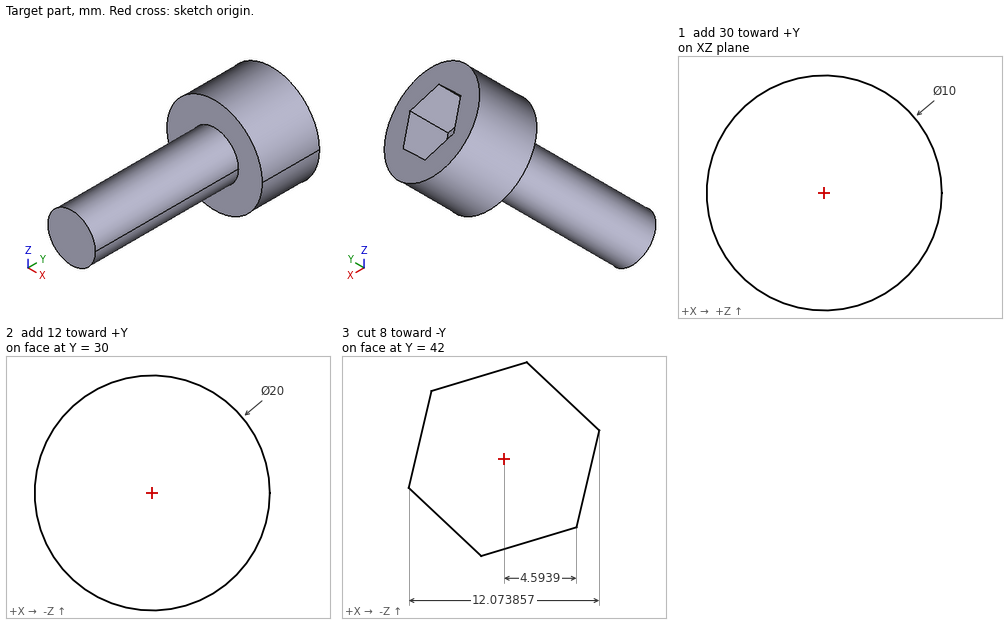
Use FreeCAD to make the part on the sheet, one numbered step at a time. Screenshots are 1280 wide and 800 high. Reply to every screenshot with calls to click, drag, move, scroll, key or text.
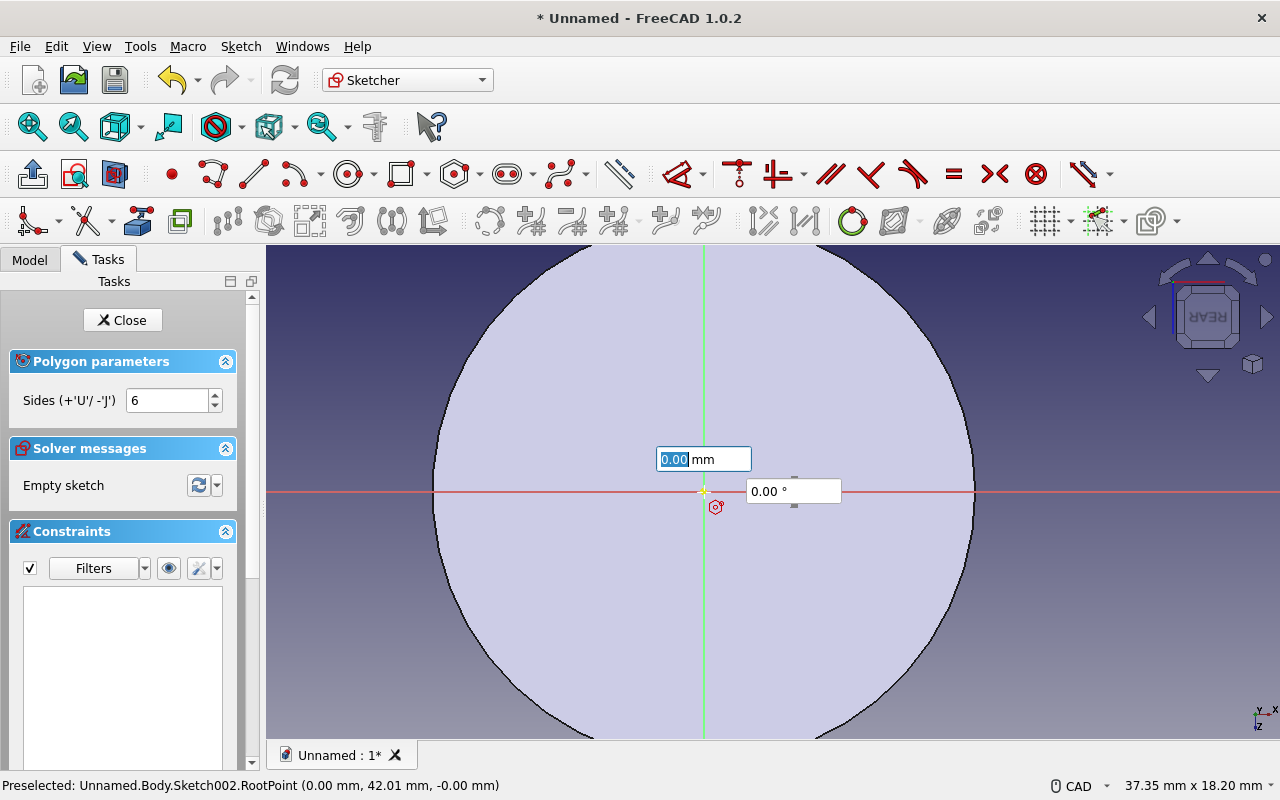
click(829, 609)
right_click(829, 609)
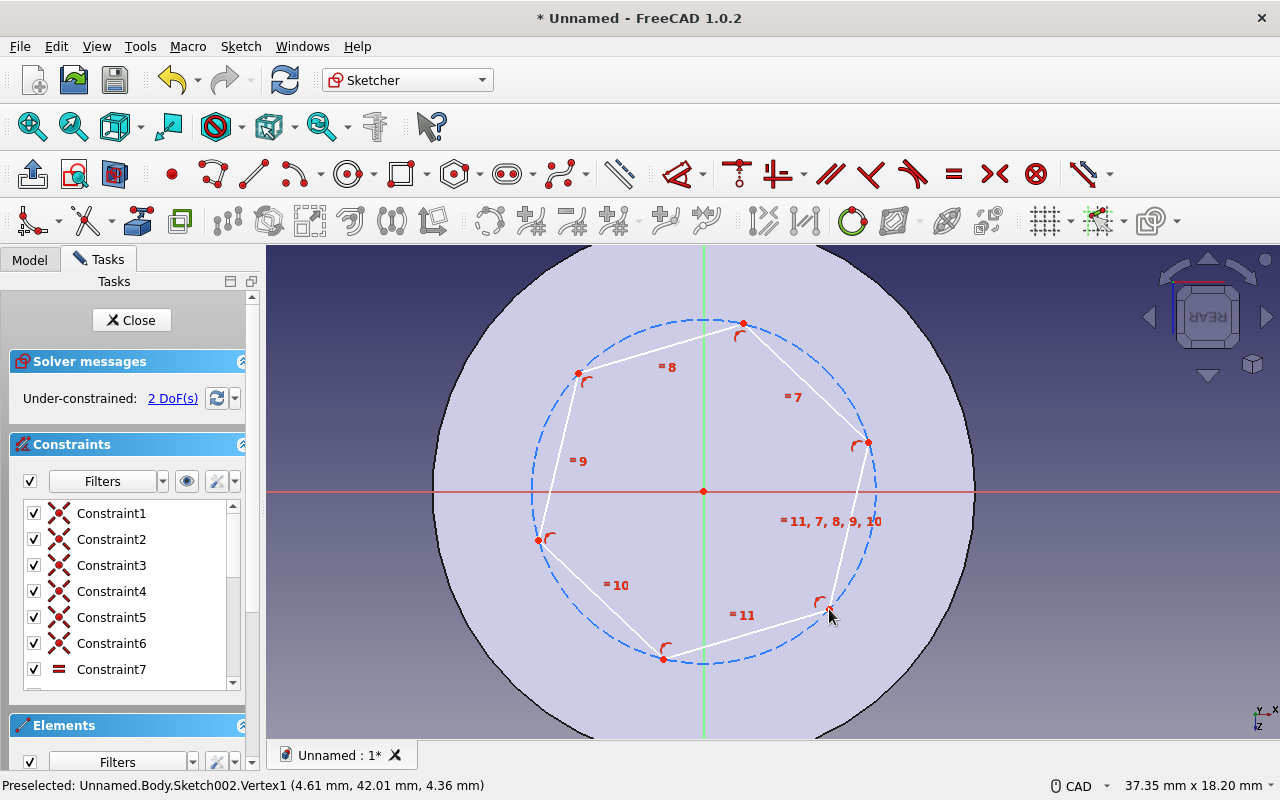
key(d)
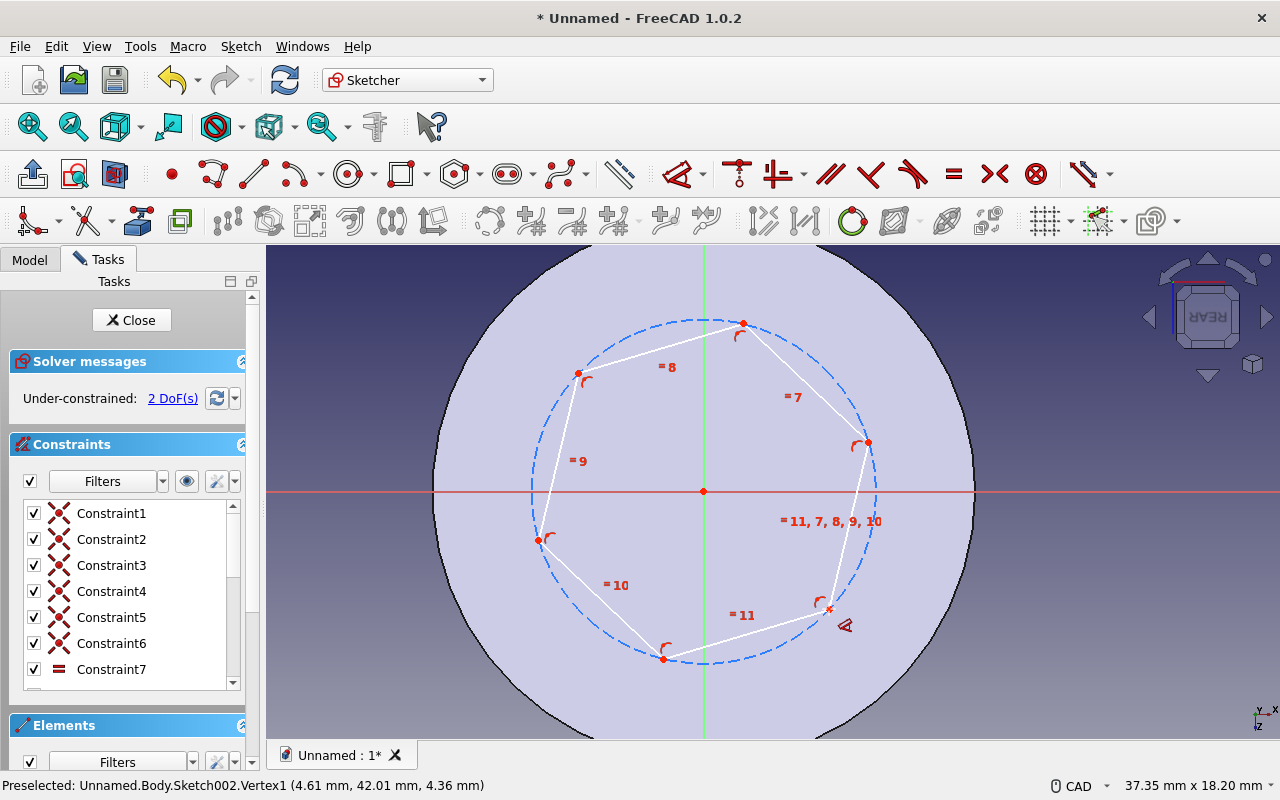
click(829, 610)
click(810, 644)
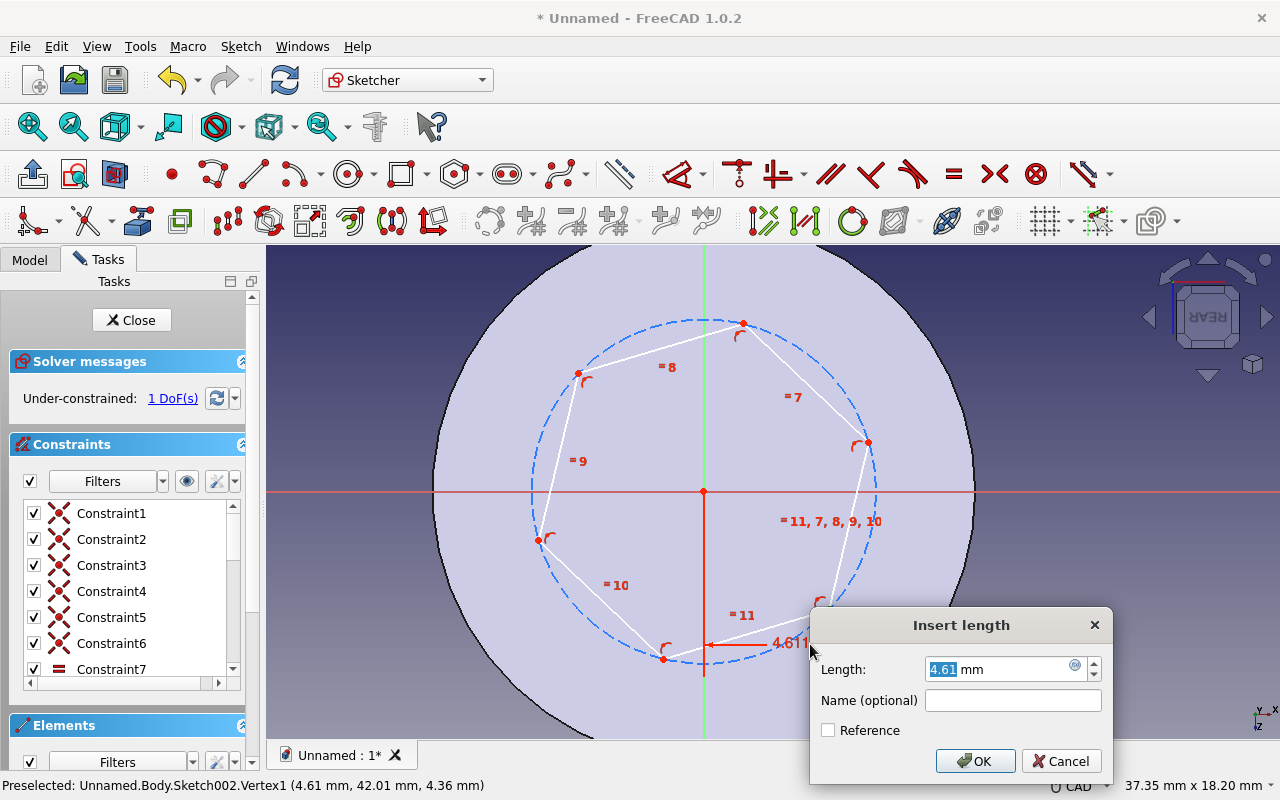
text(4.5939)
key(Return)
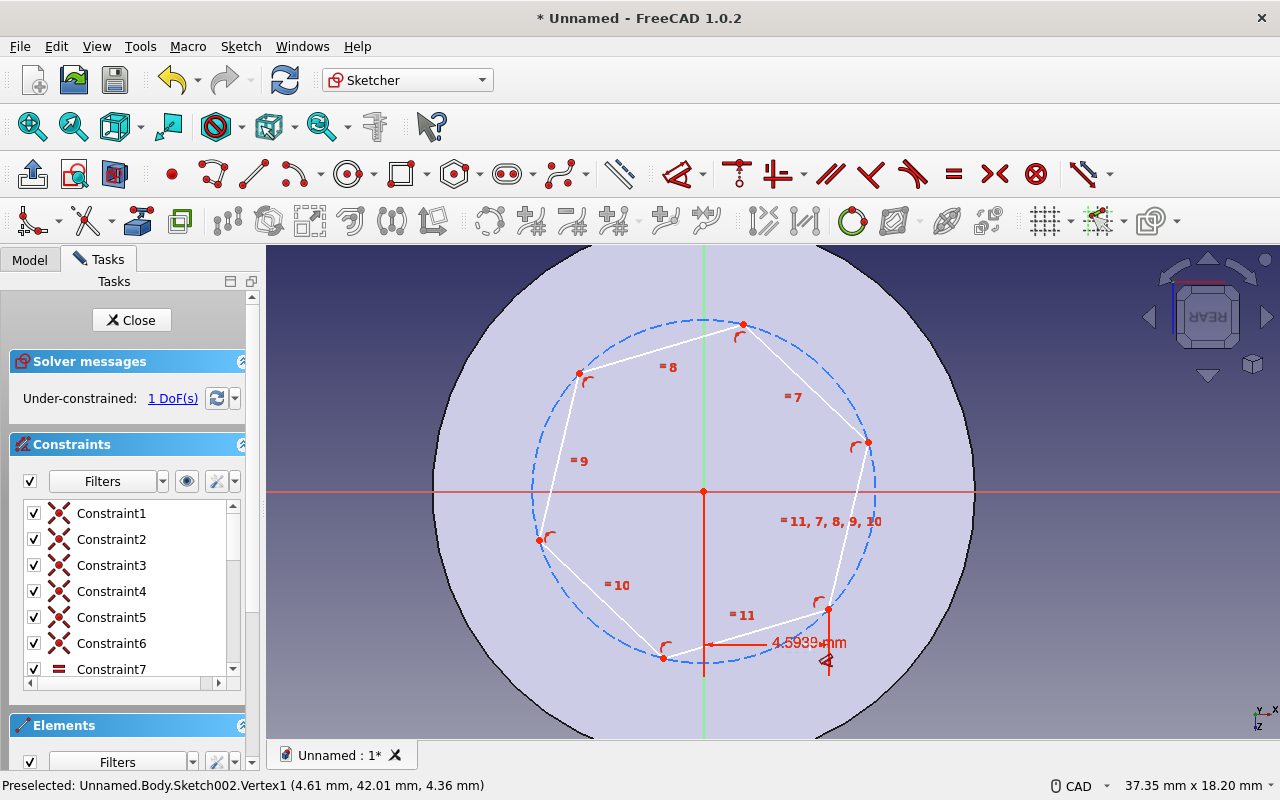
click(539, 541)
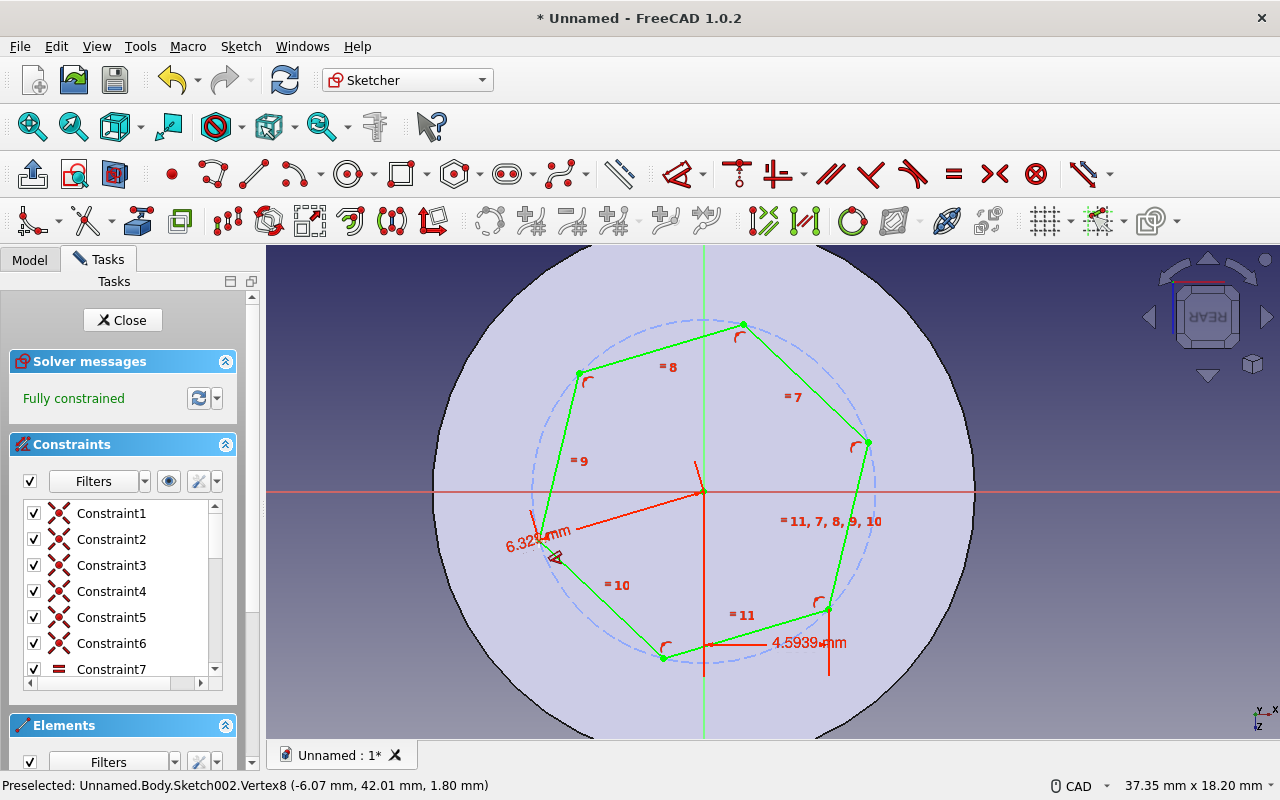
click(868, 443)
click(628, 575)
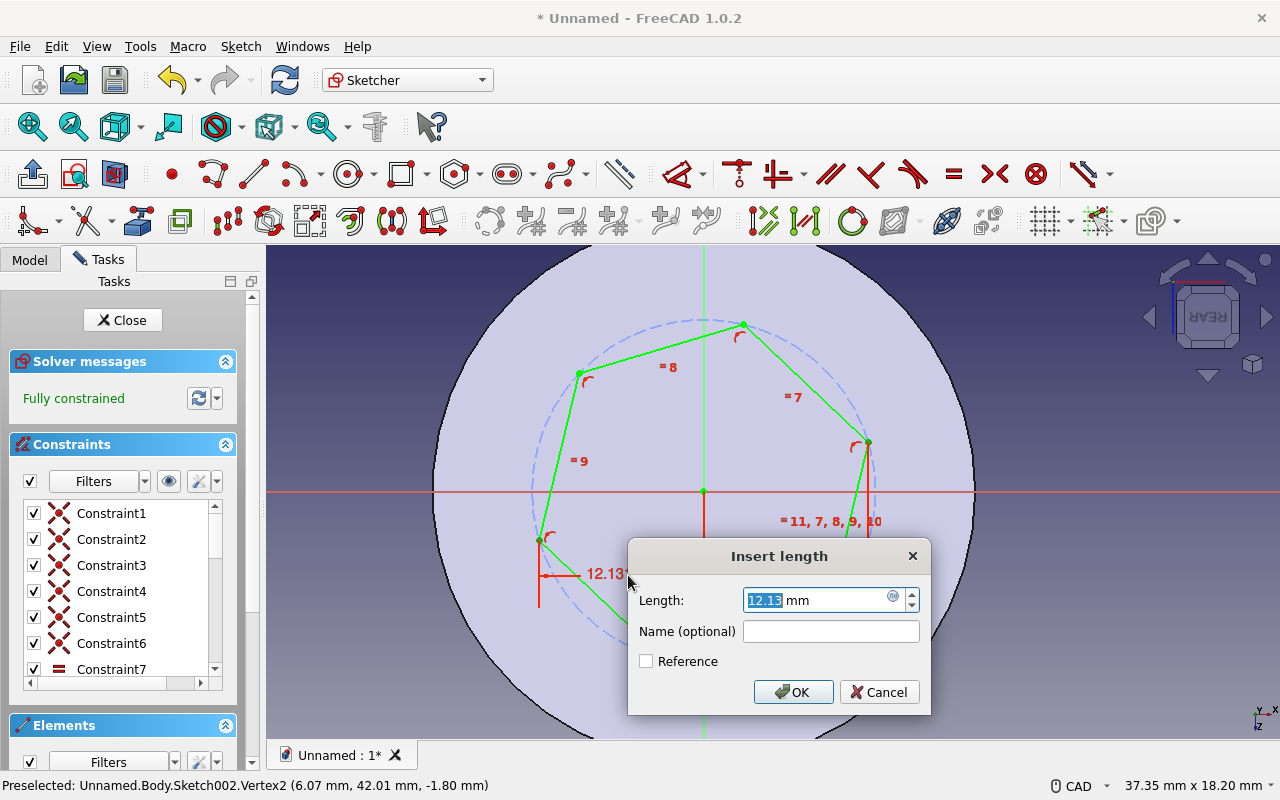
text(12.073857)
key(Return)
key(Escape)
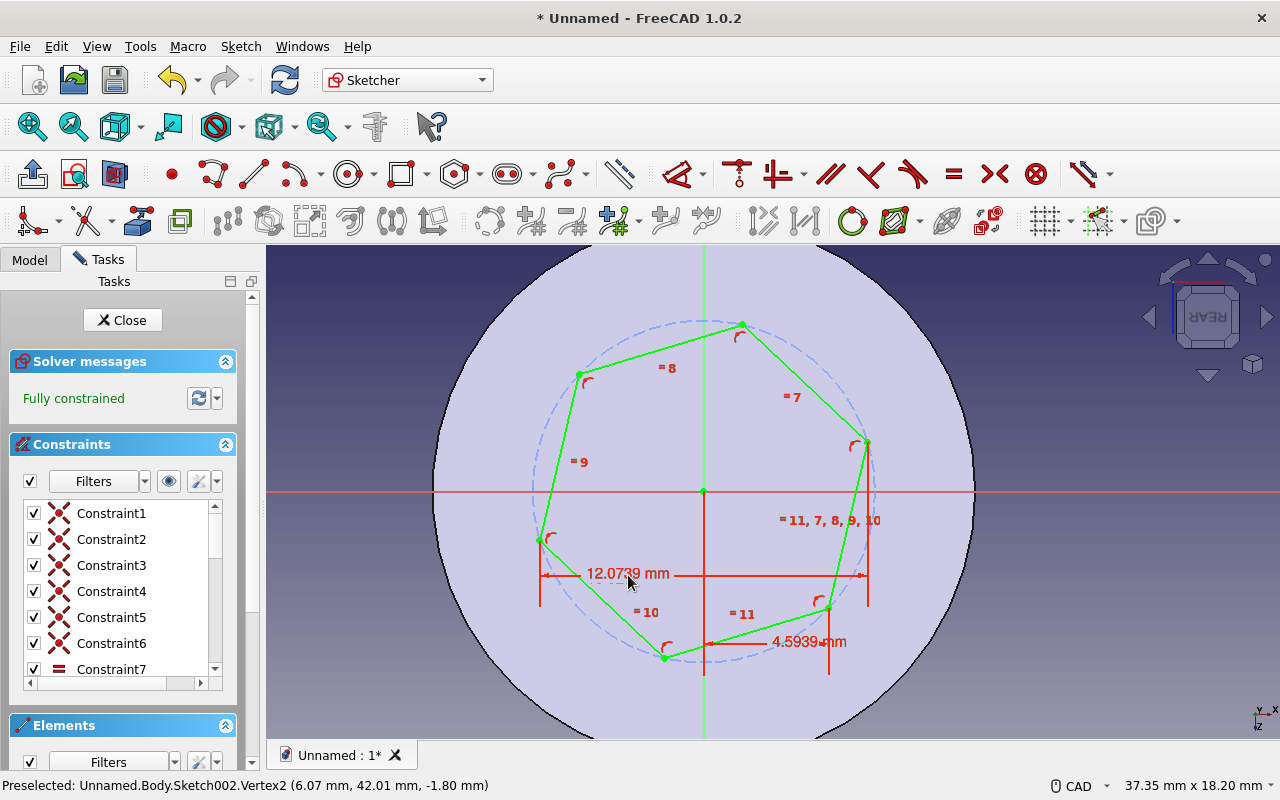
click(123, 320)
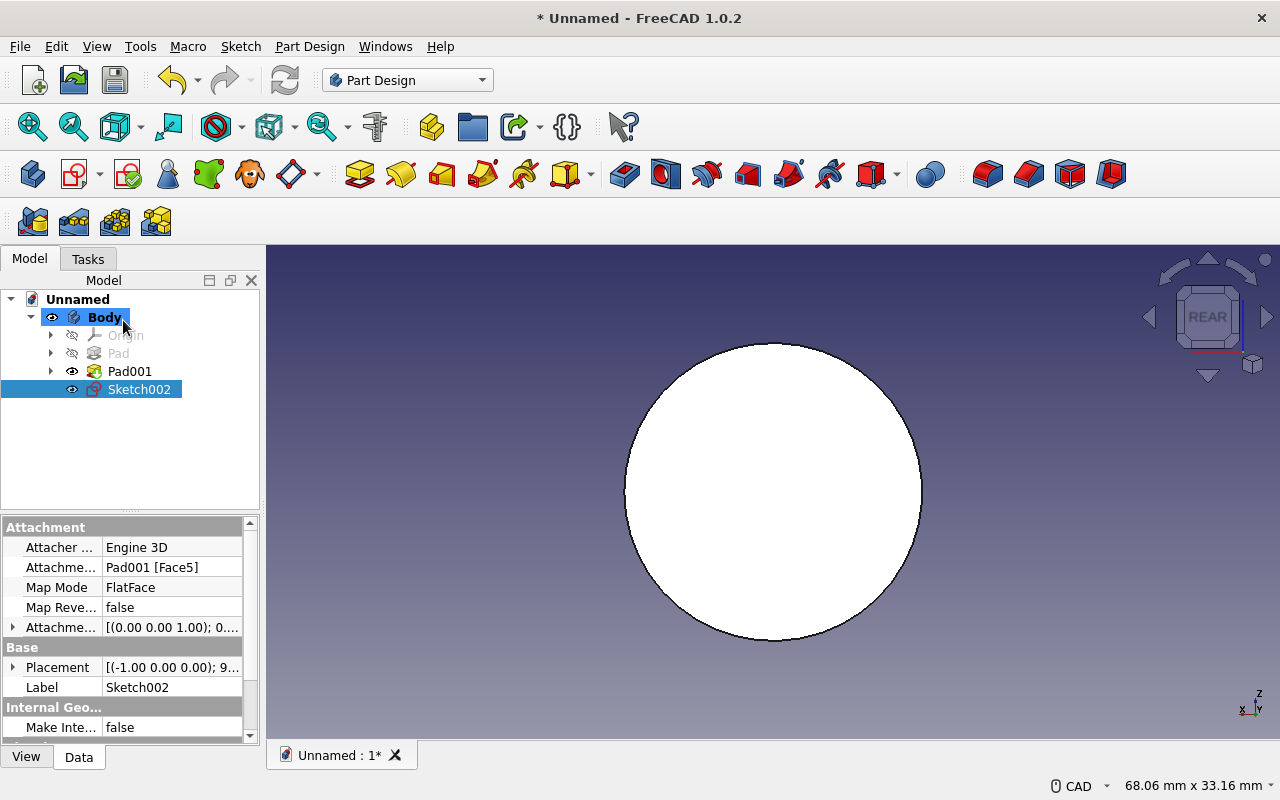
click(625, 174)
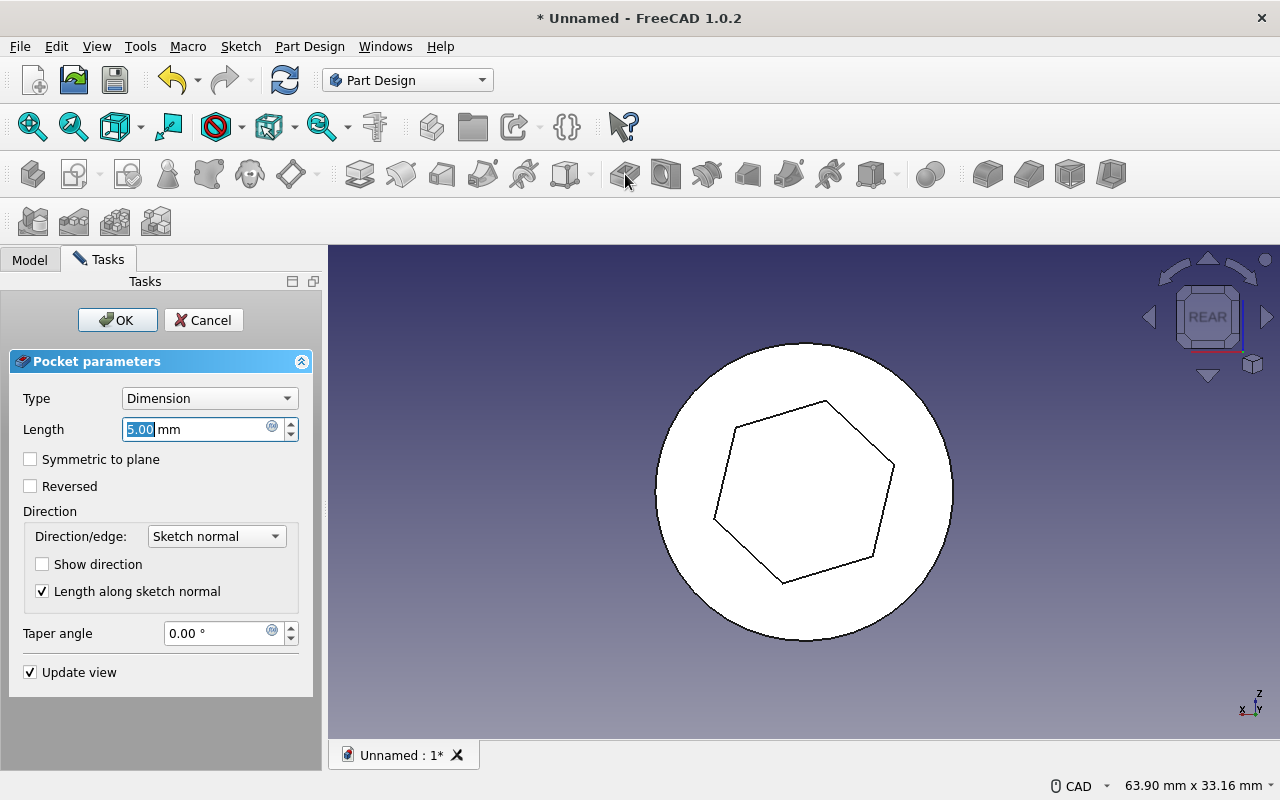
text(8)
key(Tab)